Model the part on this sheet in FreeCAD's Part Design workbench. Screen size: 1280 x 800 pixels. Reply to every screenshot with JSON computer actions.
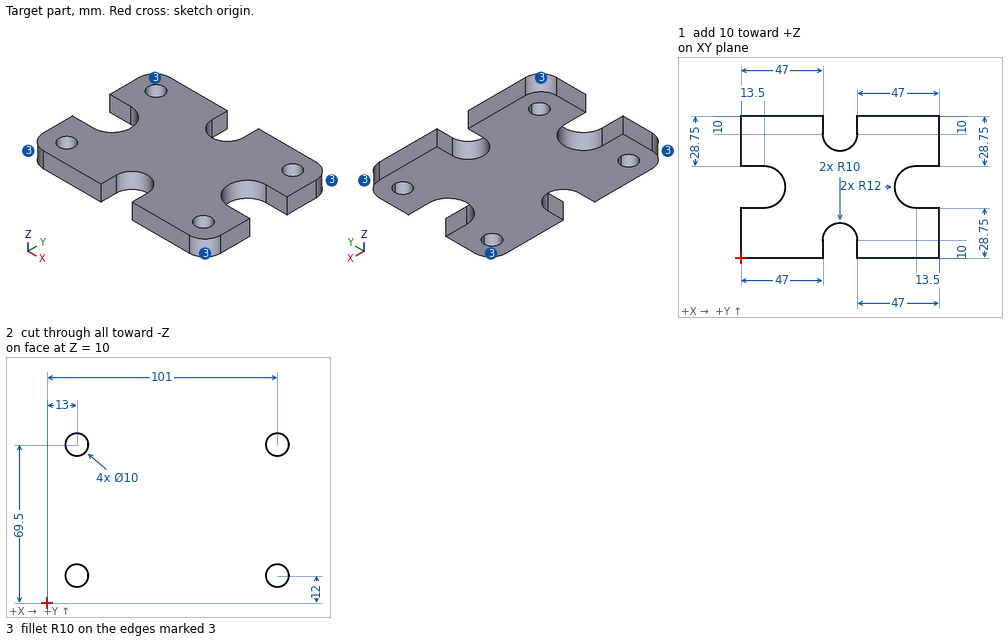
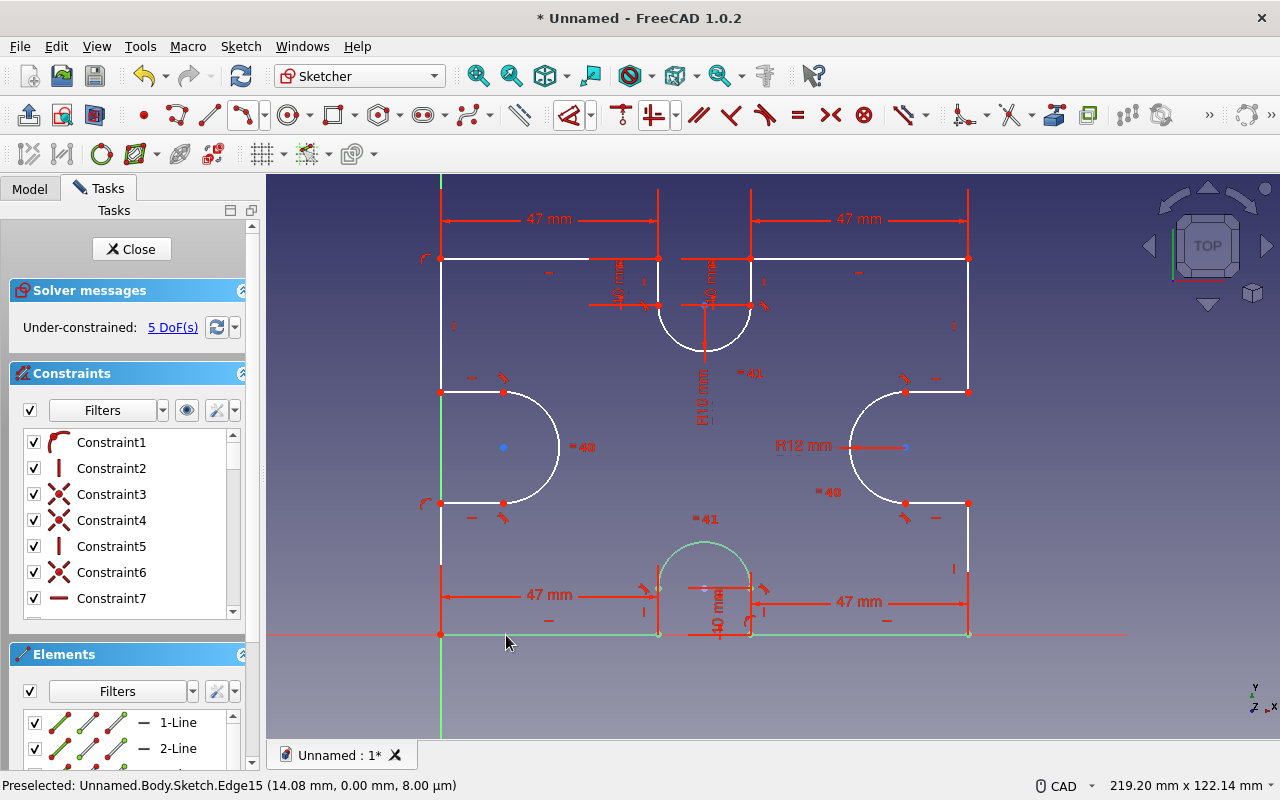
{"action": "left_click", "coordinate": [949, 503]}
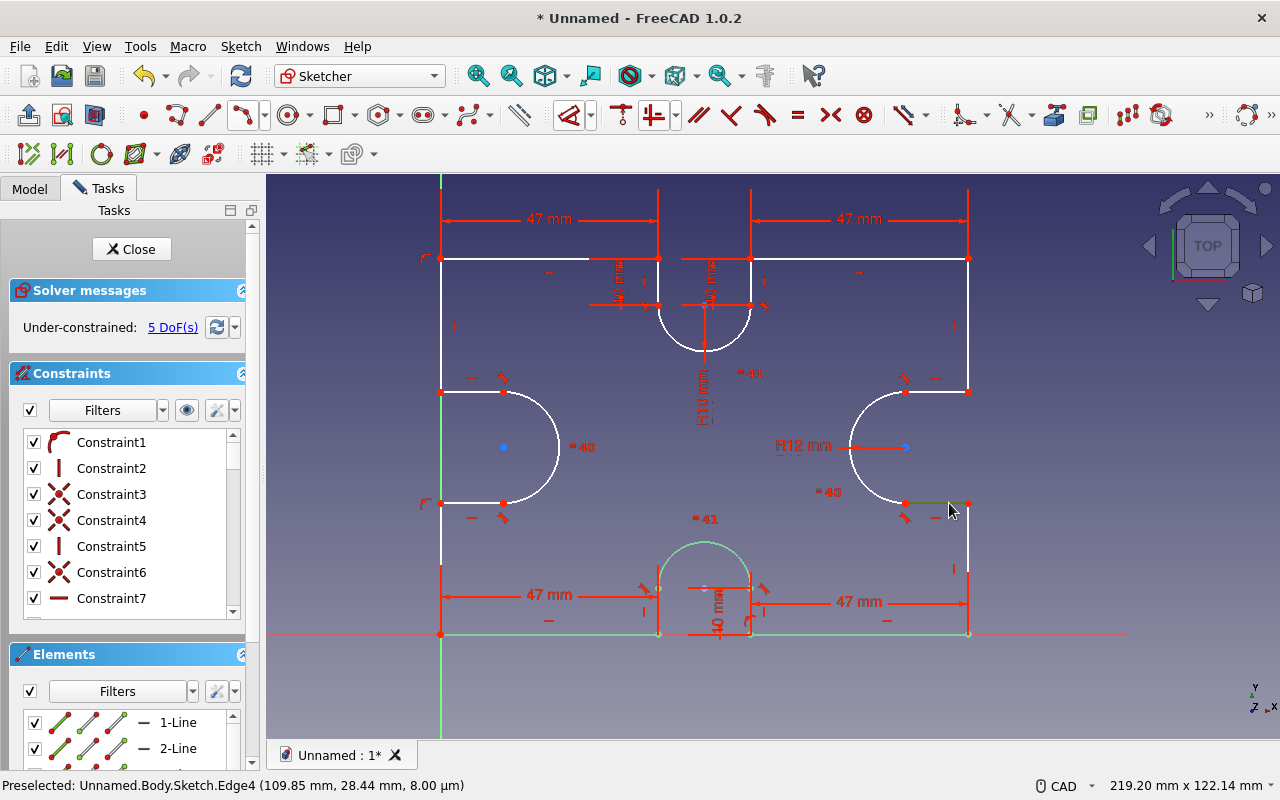
{"action": "key", "text": "l"}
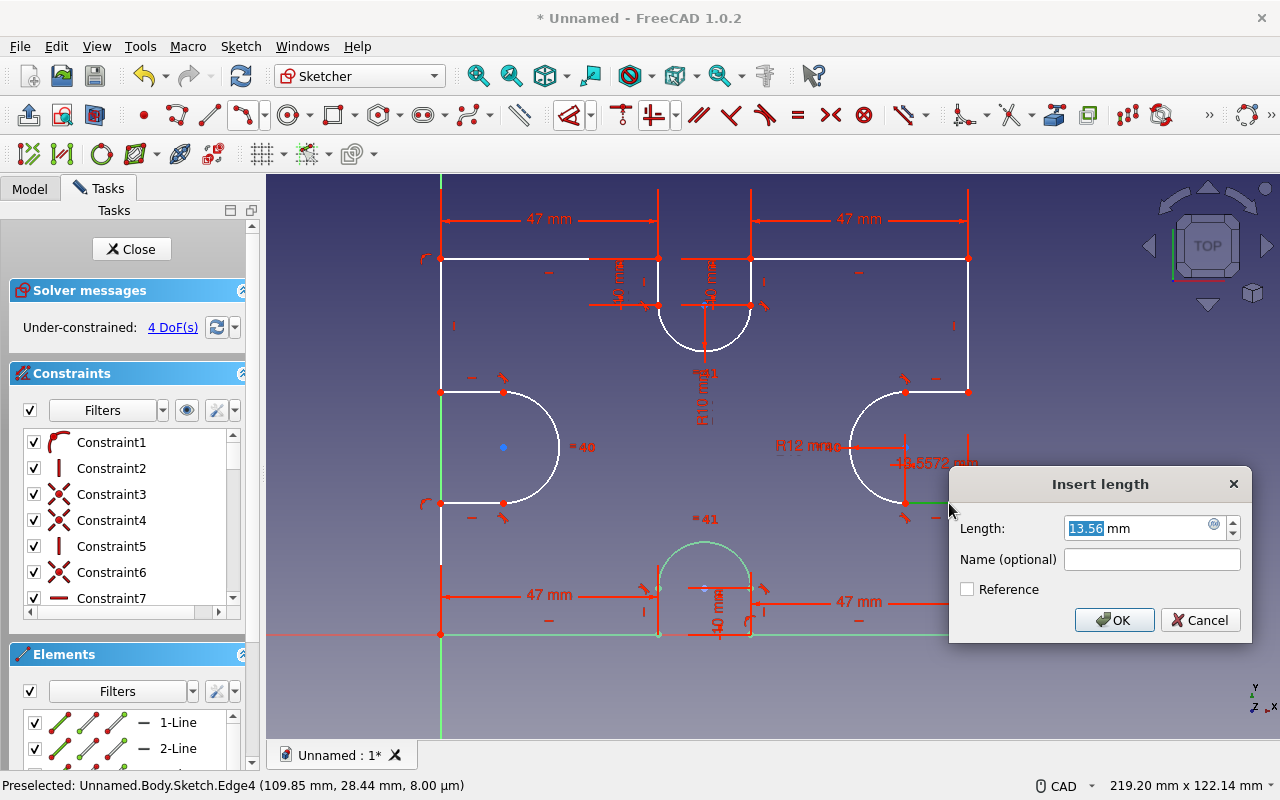
{"action": "type", "text": "13.5"}
{"action": "key", "text": "Return"}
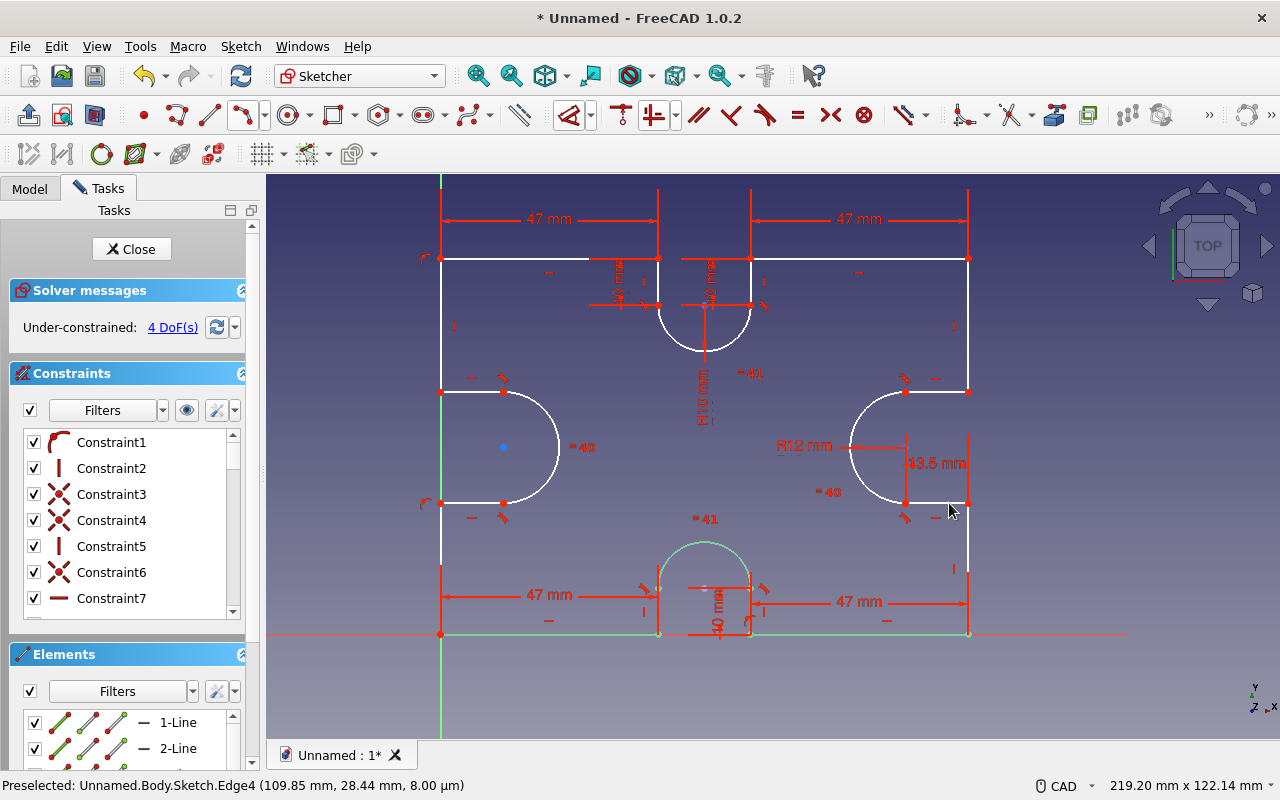
{"action": "left_click", "coordinate": [460, 392]}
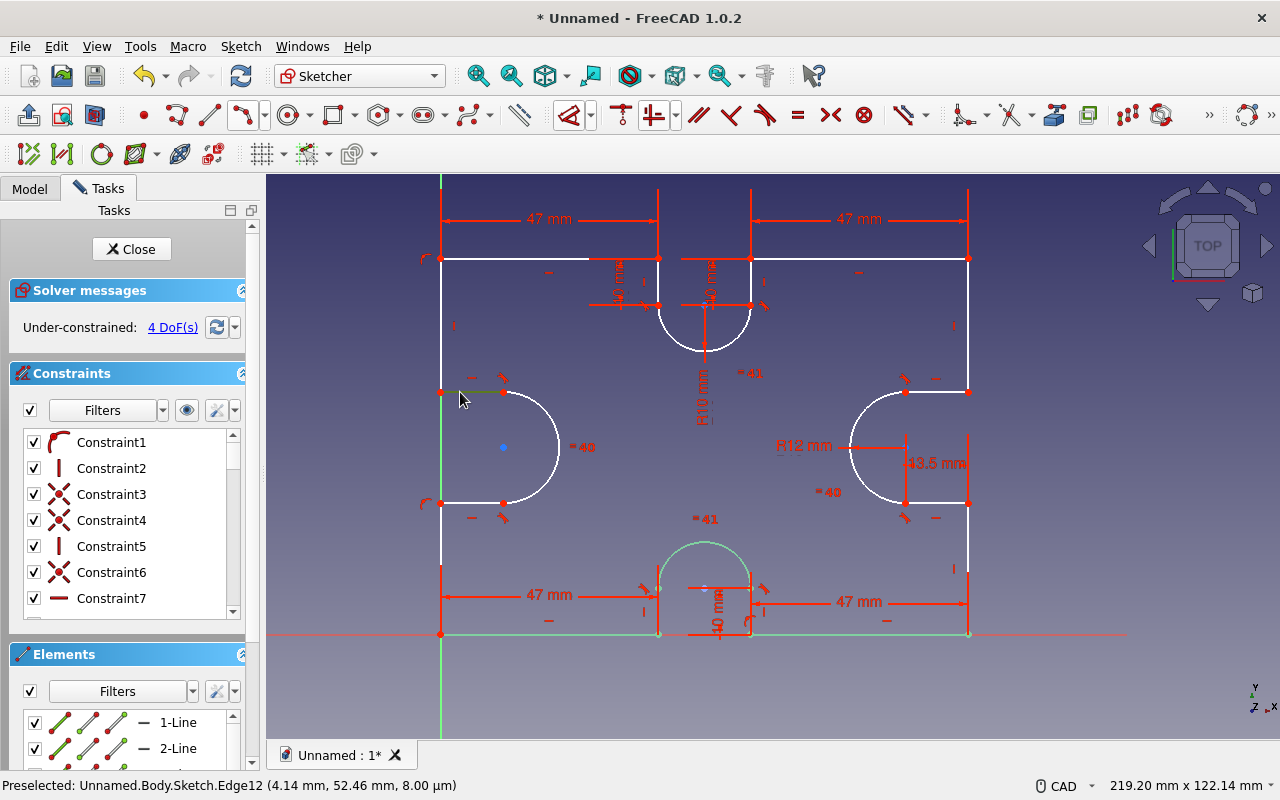
{"action": "key", "text": "l"}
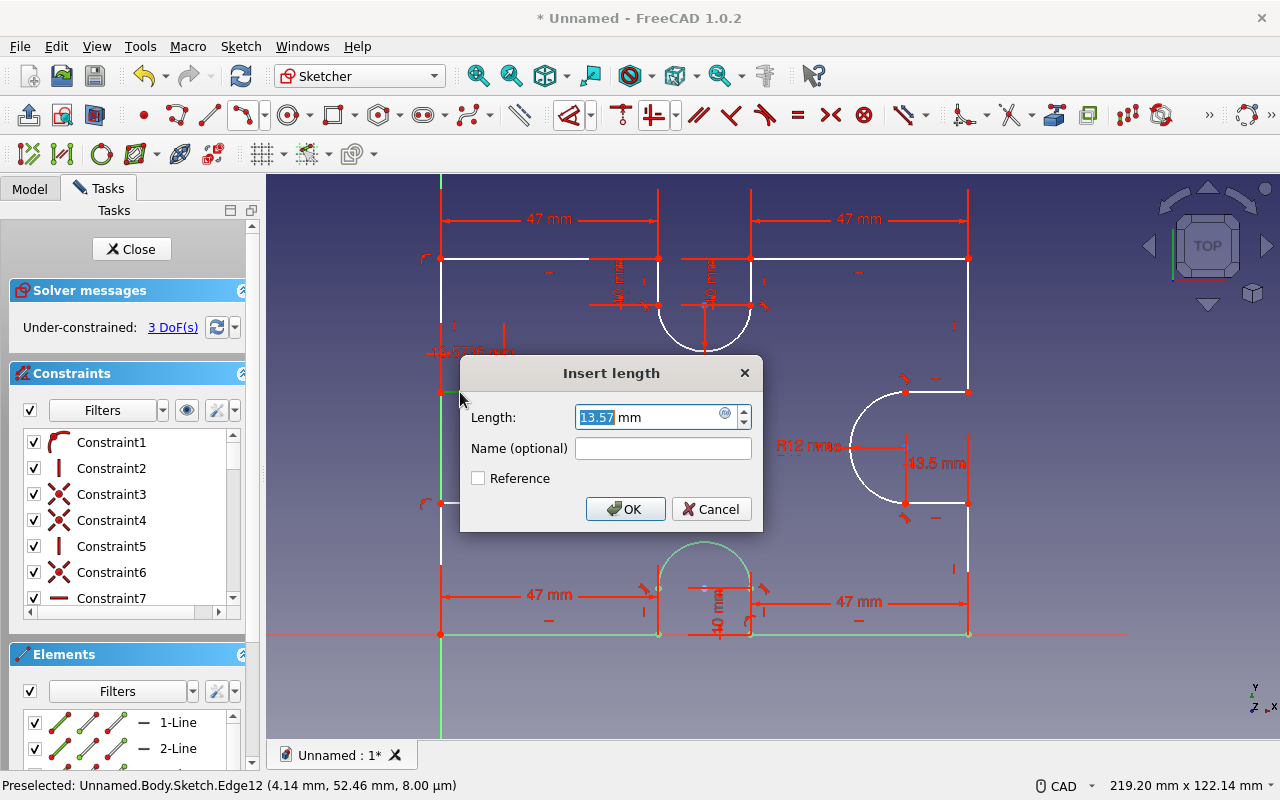
{"action": "type", "text": "13.5"}
{"action": "key", "text": "Return"}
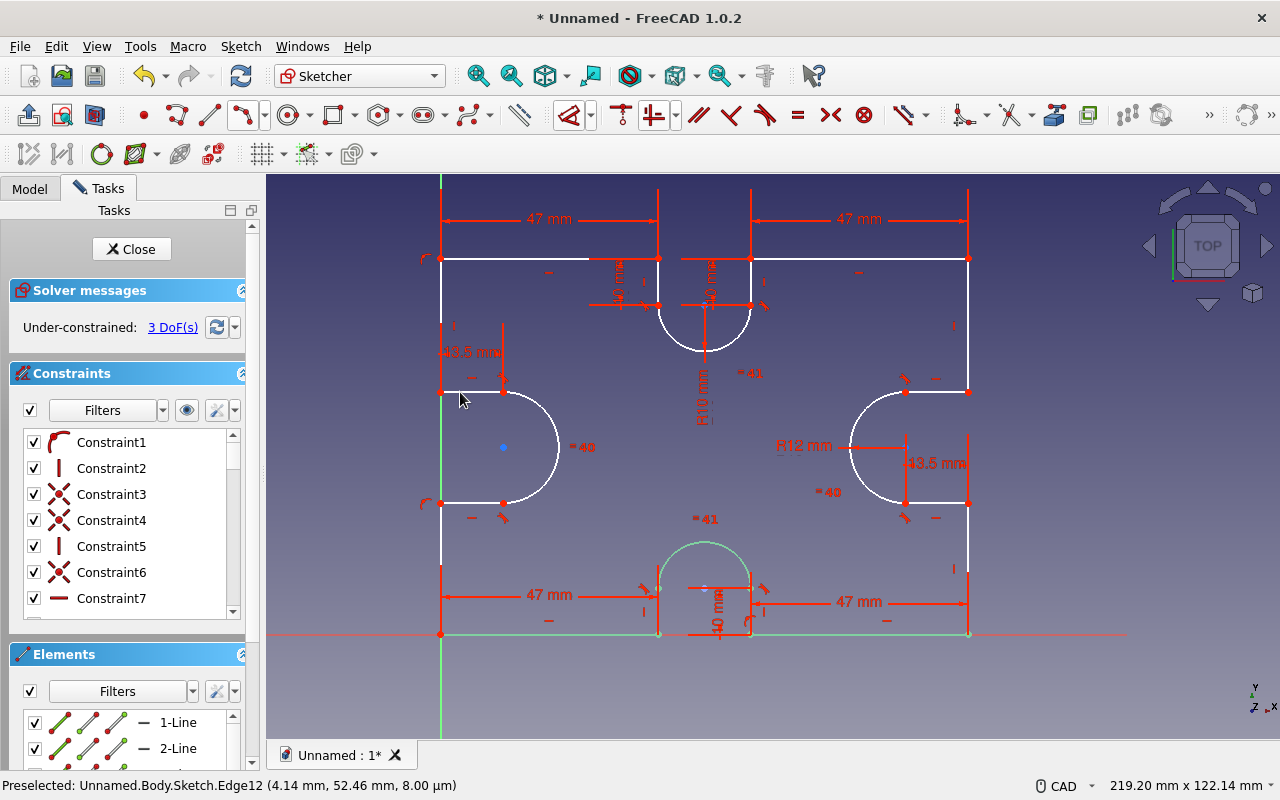
{"action": "left_click", "coordinate": [968, 595]}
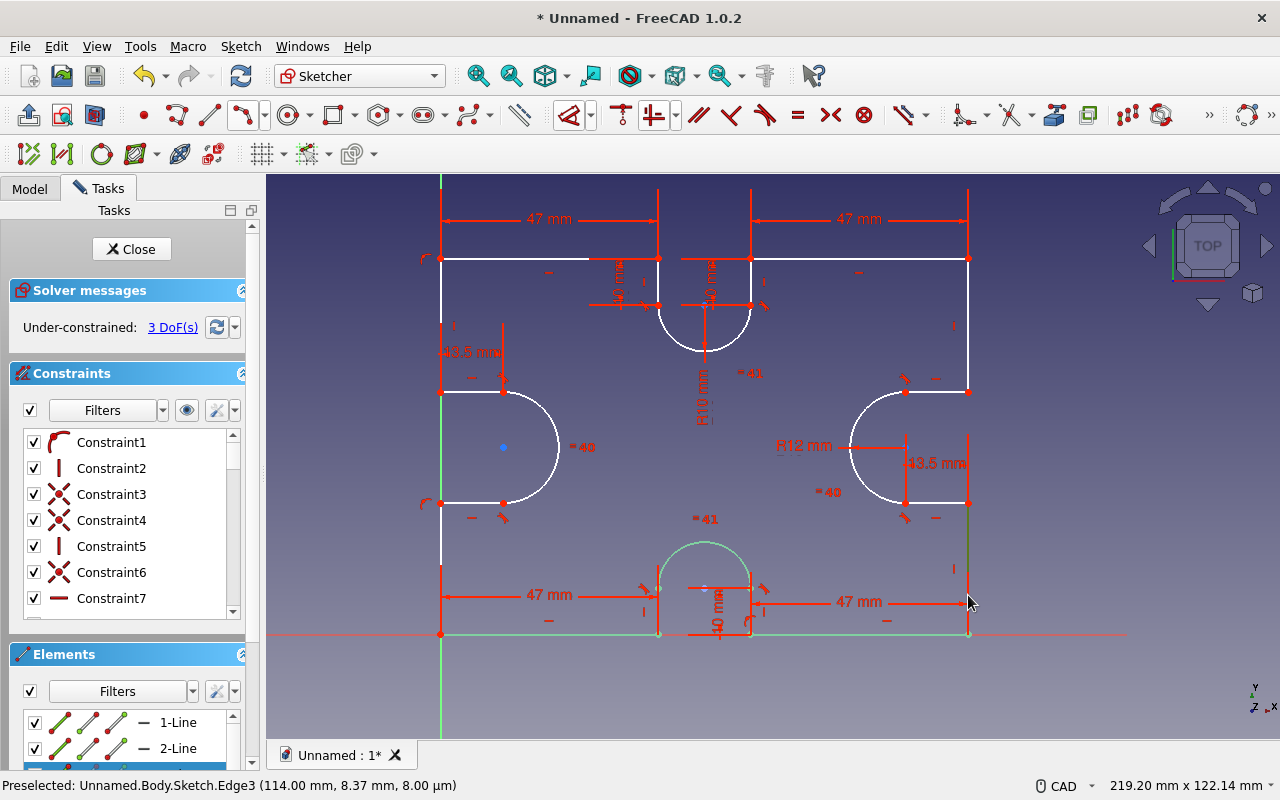
{"action": "left_click", "coordinate": [590, 116]}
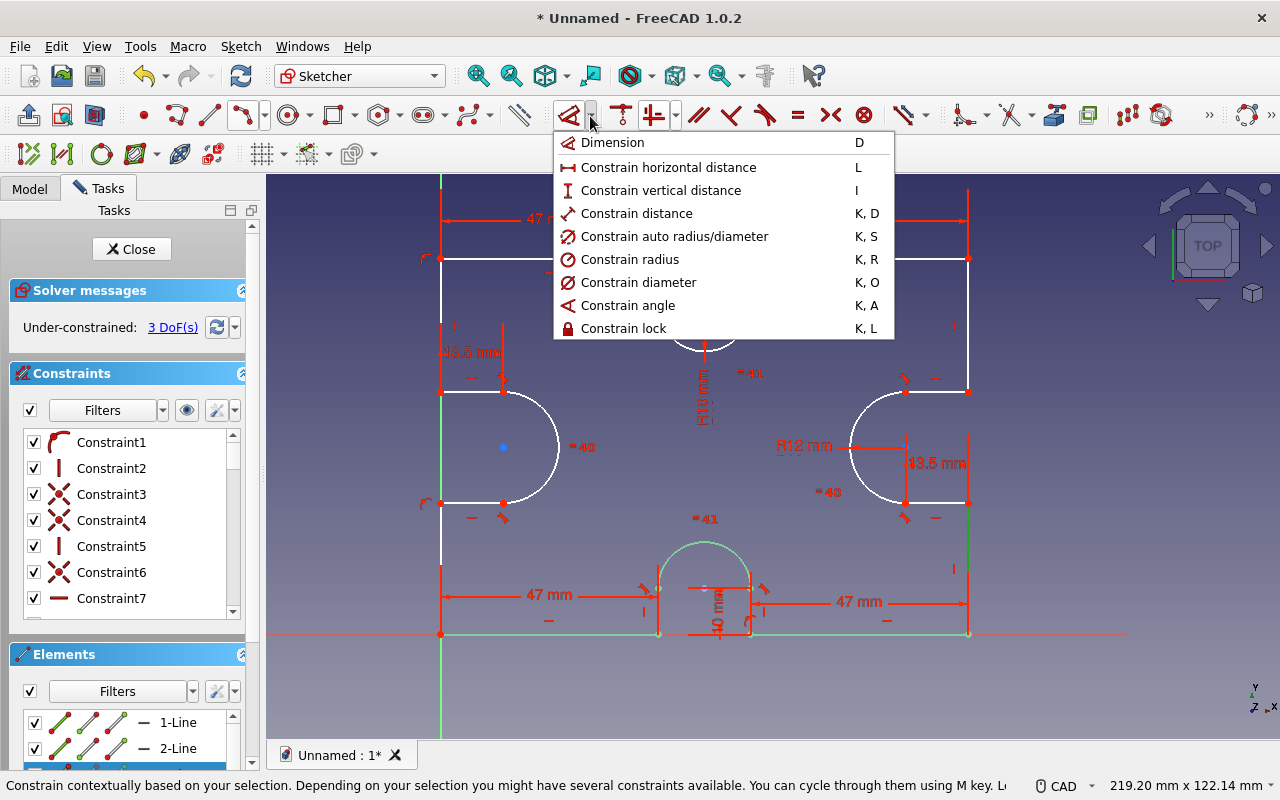
{"action": "left_click", "coordinate": [724, 190]}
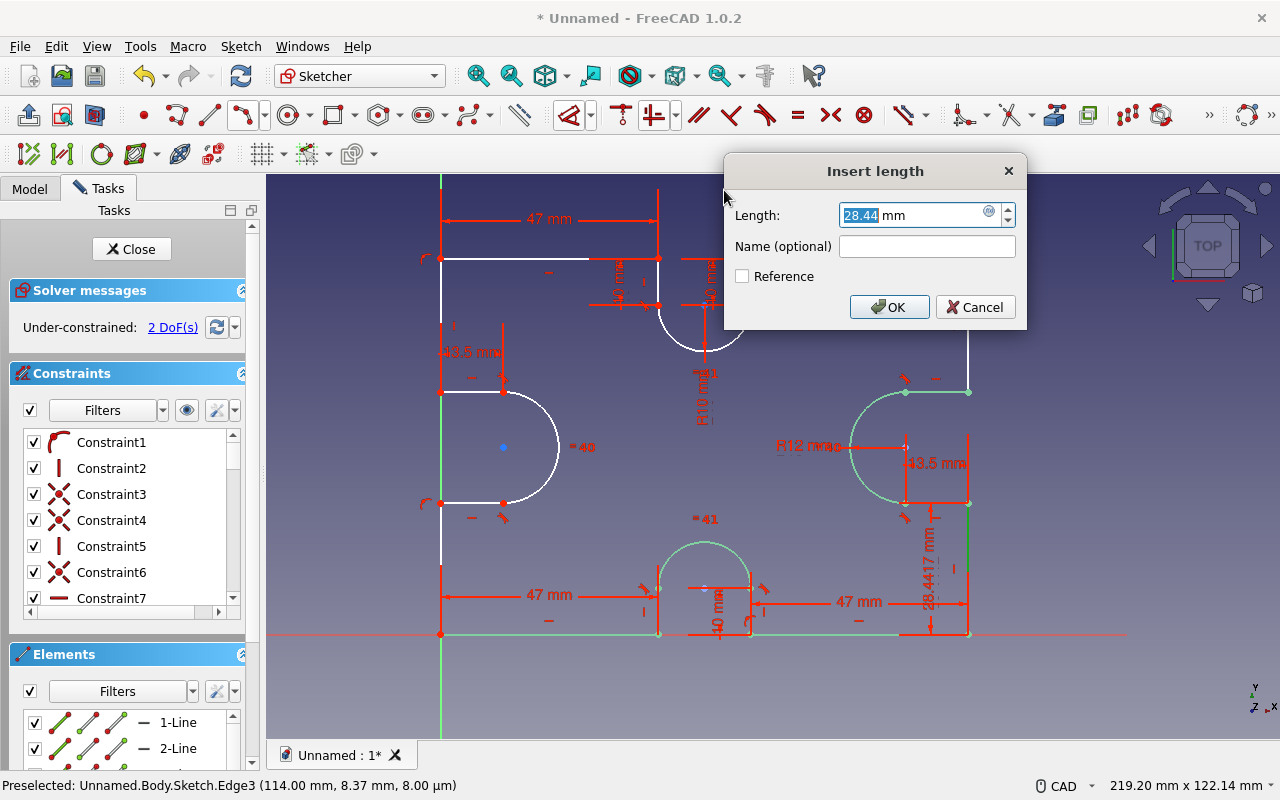
{"action": "type", "text": "28.75"}
{"action": "key", "text": "Return"}